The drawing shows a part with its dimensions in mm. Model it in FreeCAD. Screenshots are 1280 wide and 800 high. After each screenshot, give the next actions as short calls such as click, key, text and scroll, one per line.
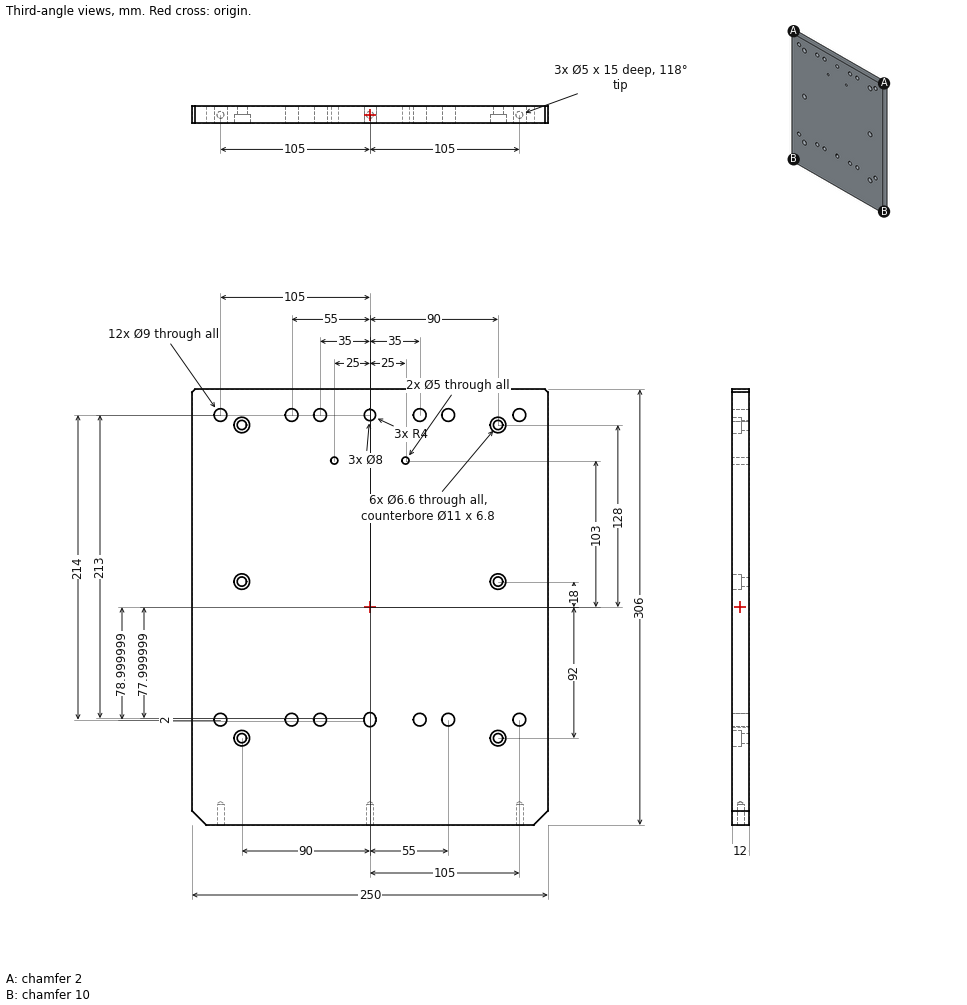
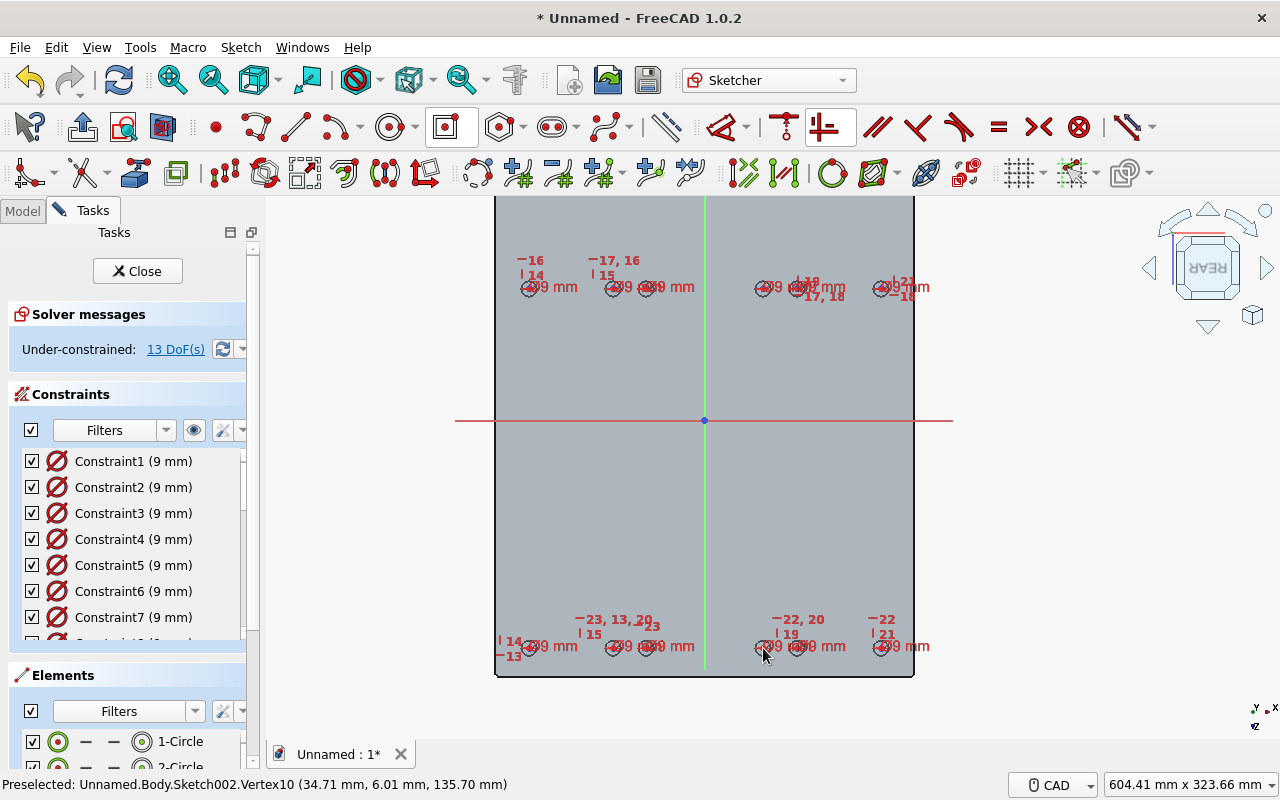
key(h)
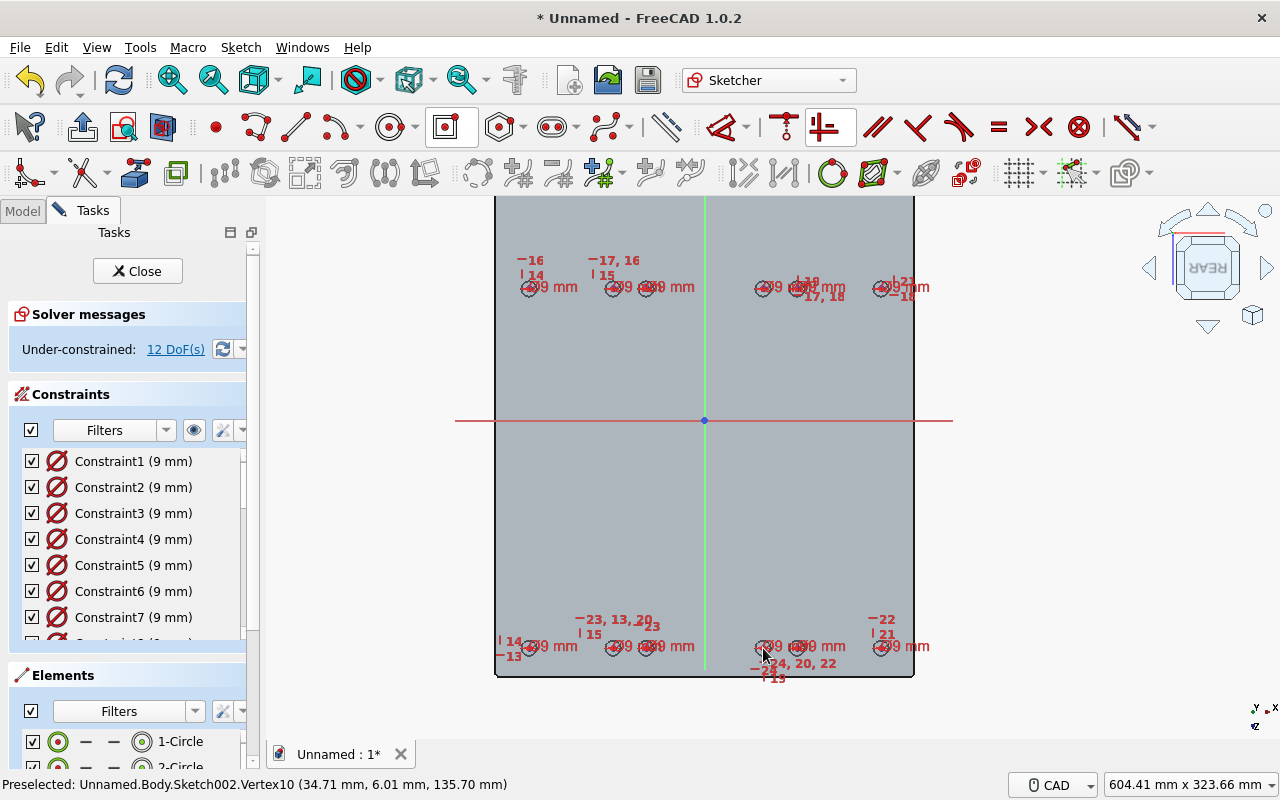
click(646, 648)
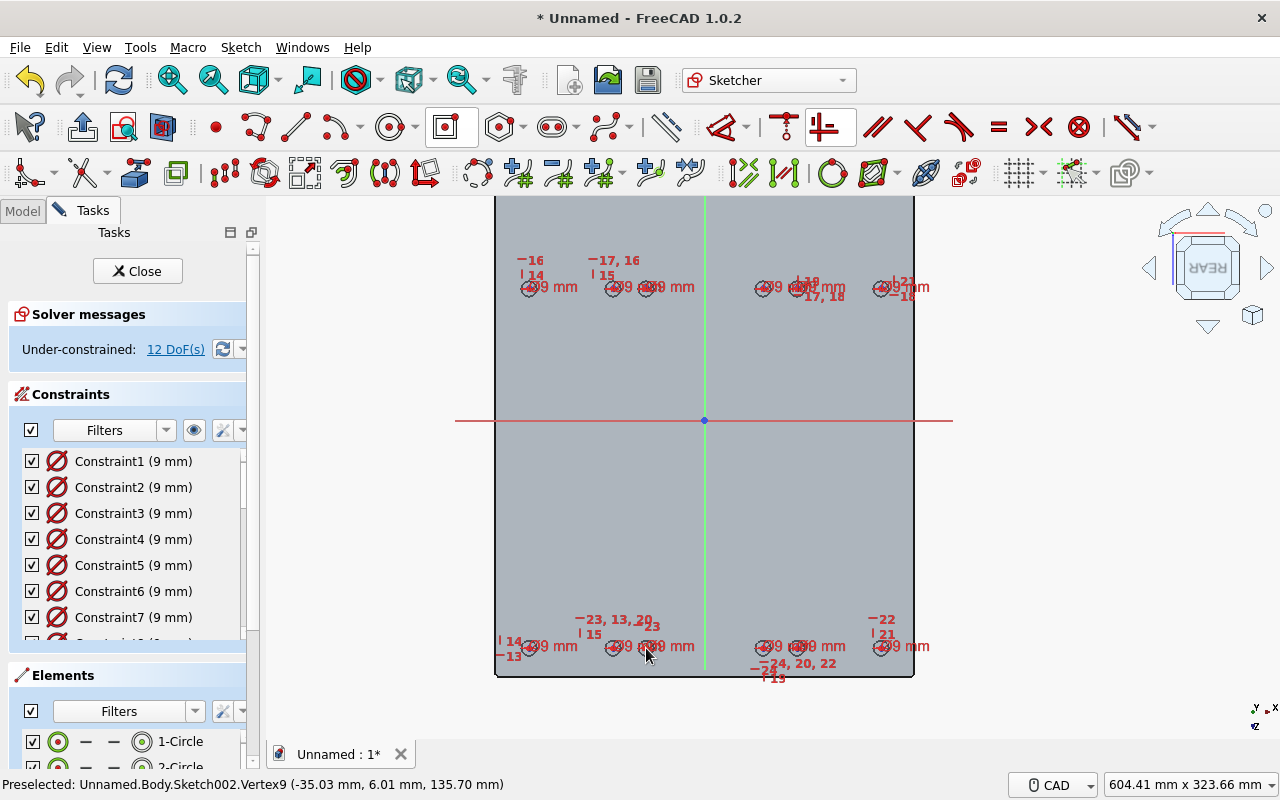
click(646, 289)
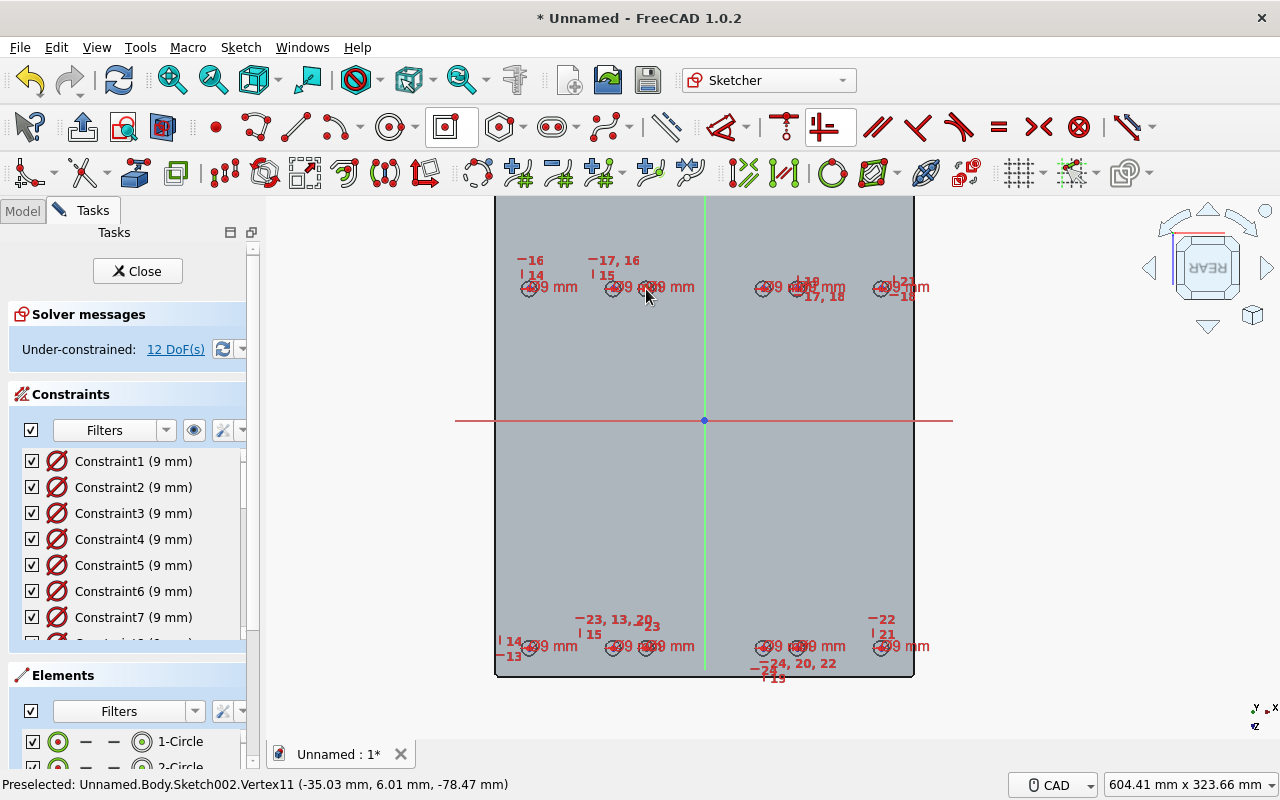
click(850, 128)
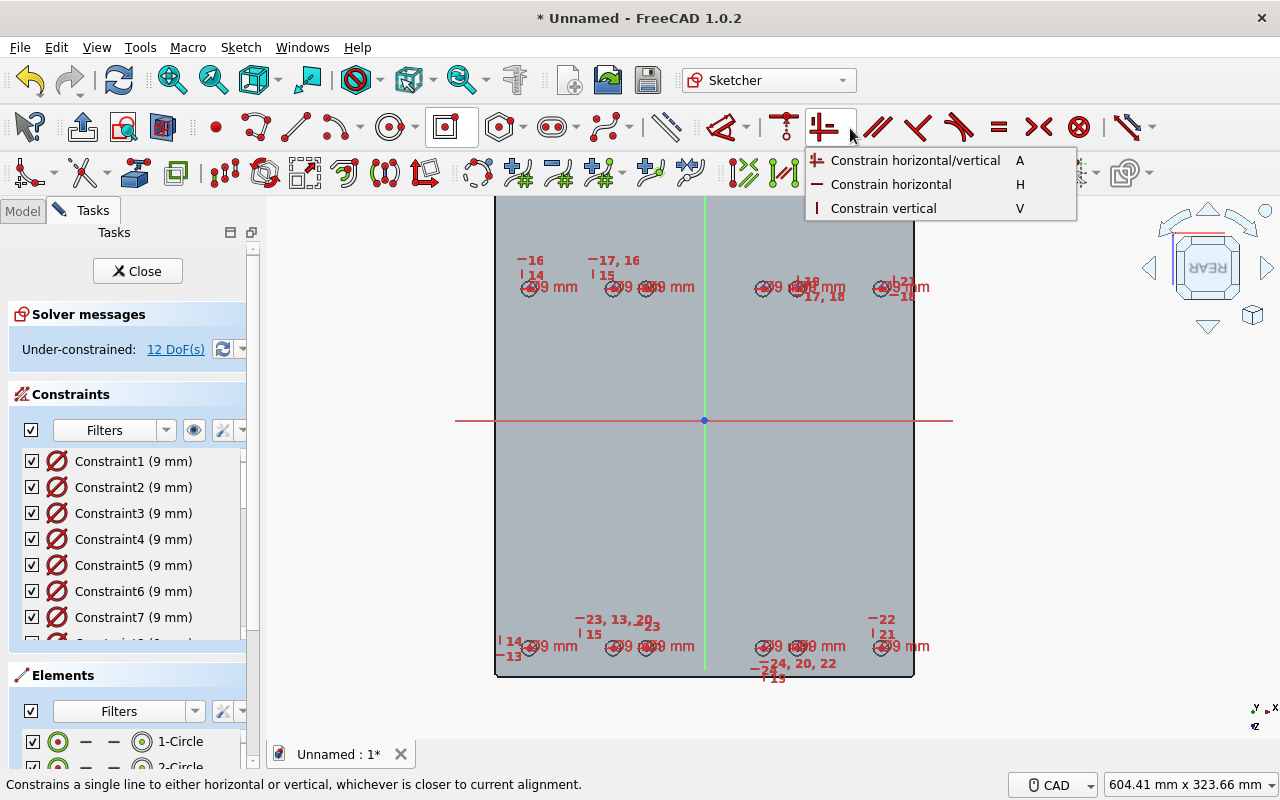
click(941, 208)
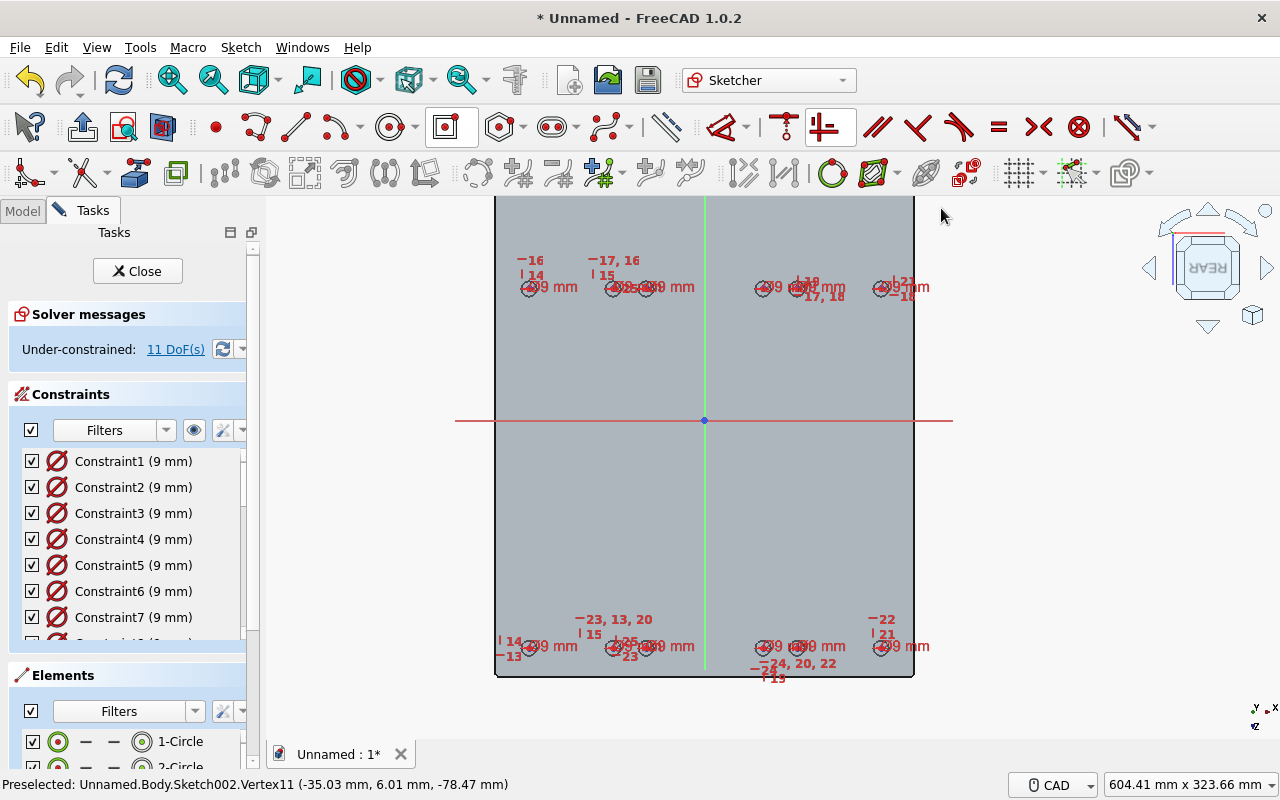
scroll(613, 289, up, 4)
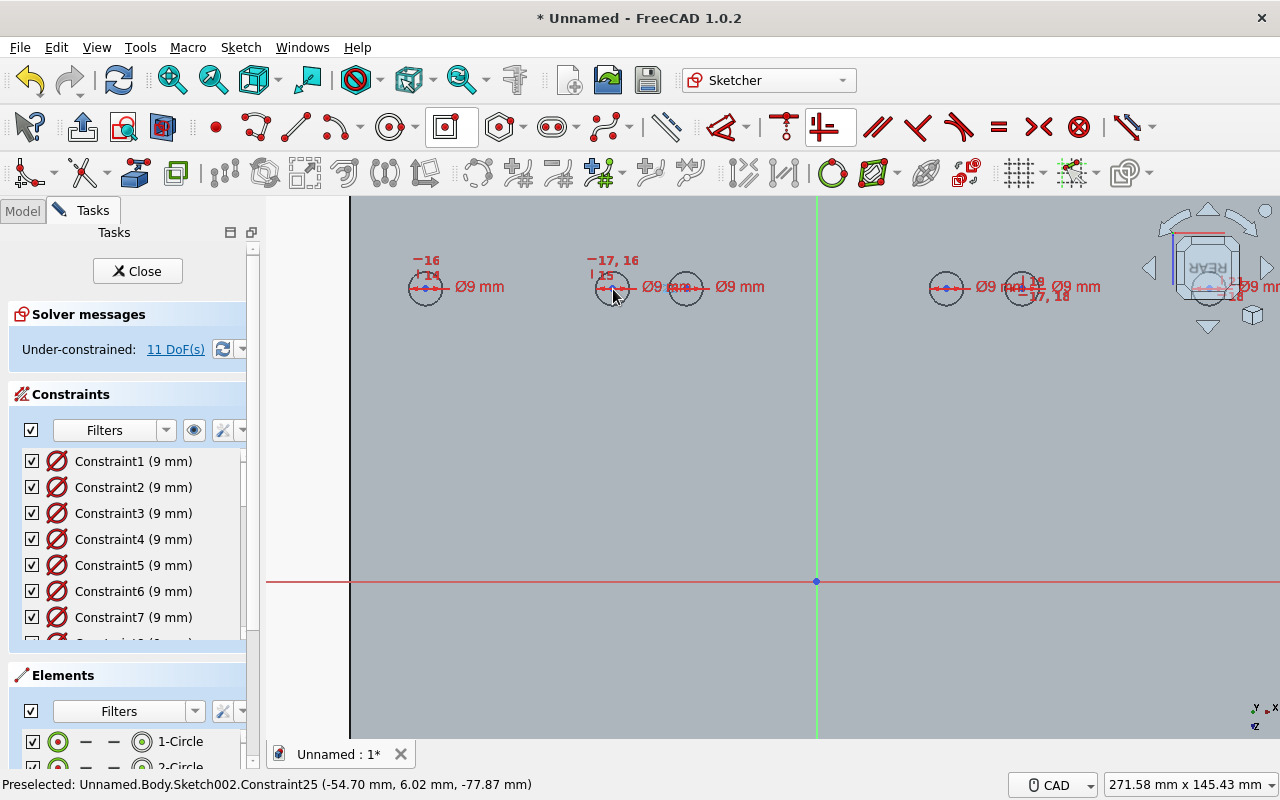
click(613, 289)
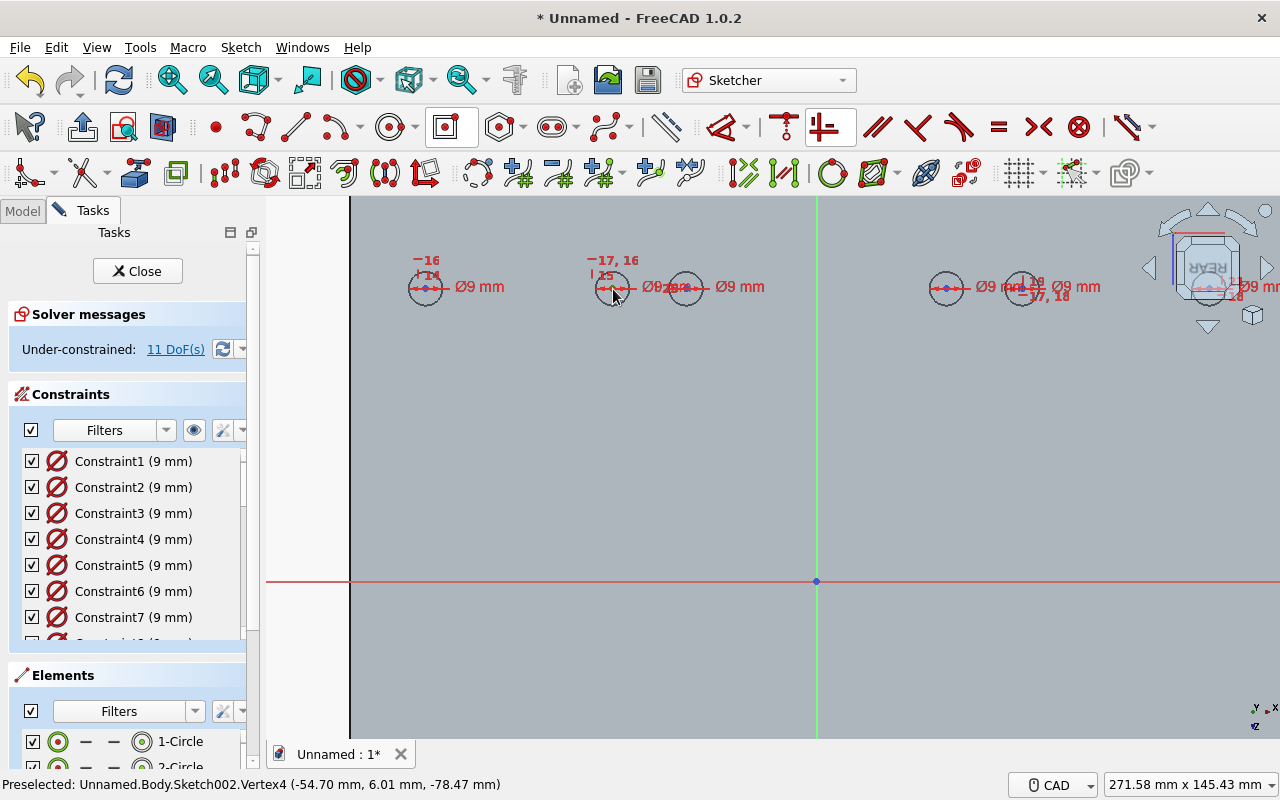
click(686, 289)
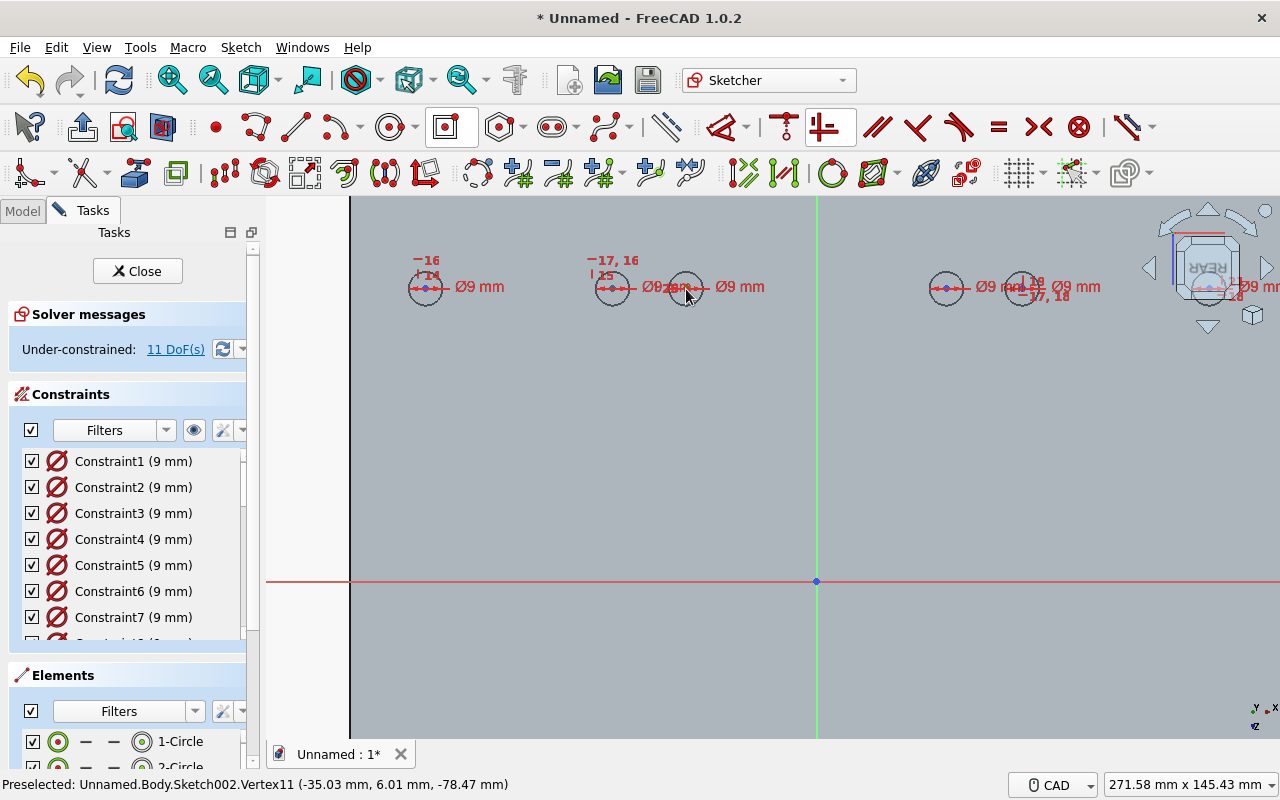
key(h)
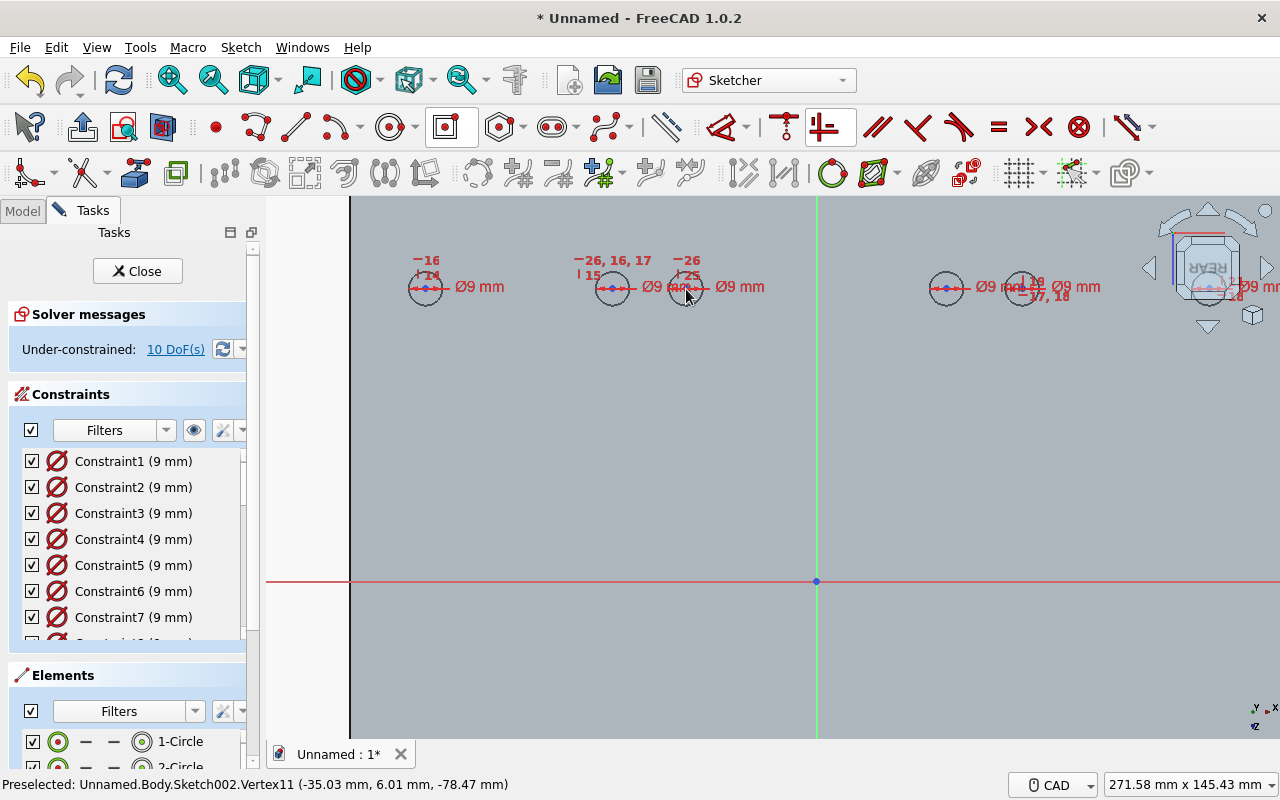
scroll(613, 289, down, 4)